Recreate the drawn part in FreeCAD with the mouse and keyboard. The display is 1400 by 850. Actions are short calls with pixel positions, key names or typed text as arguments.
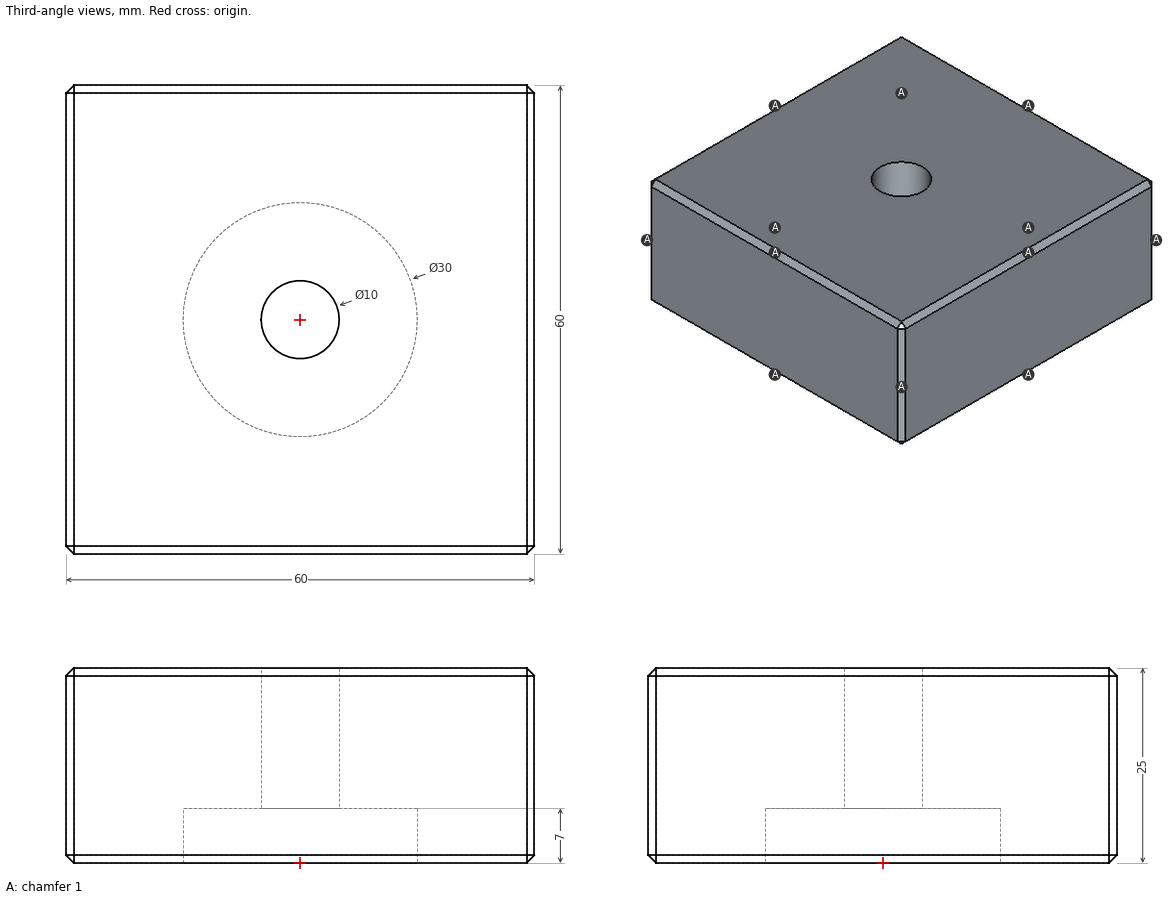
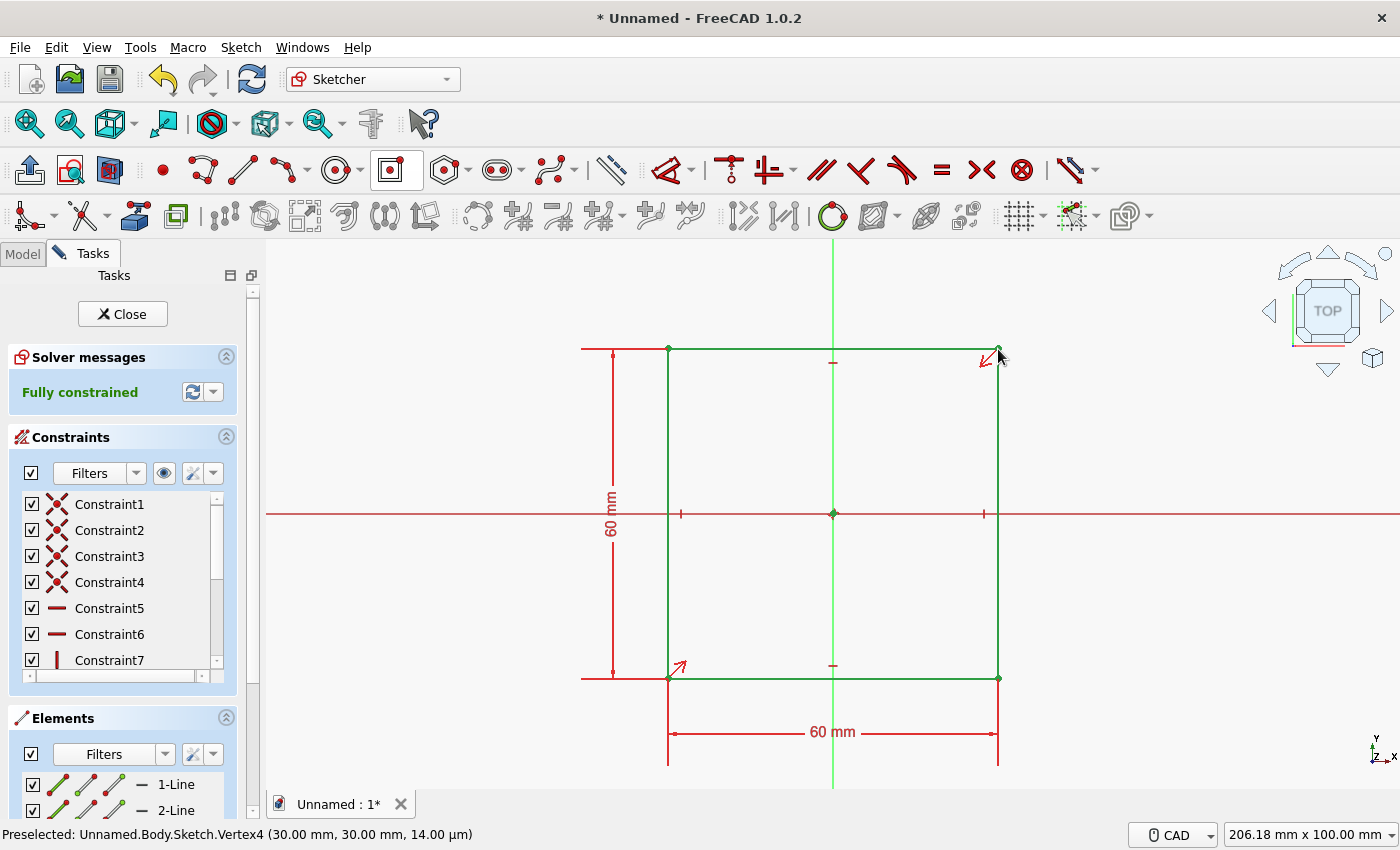
click(123, 314)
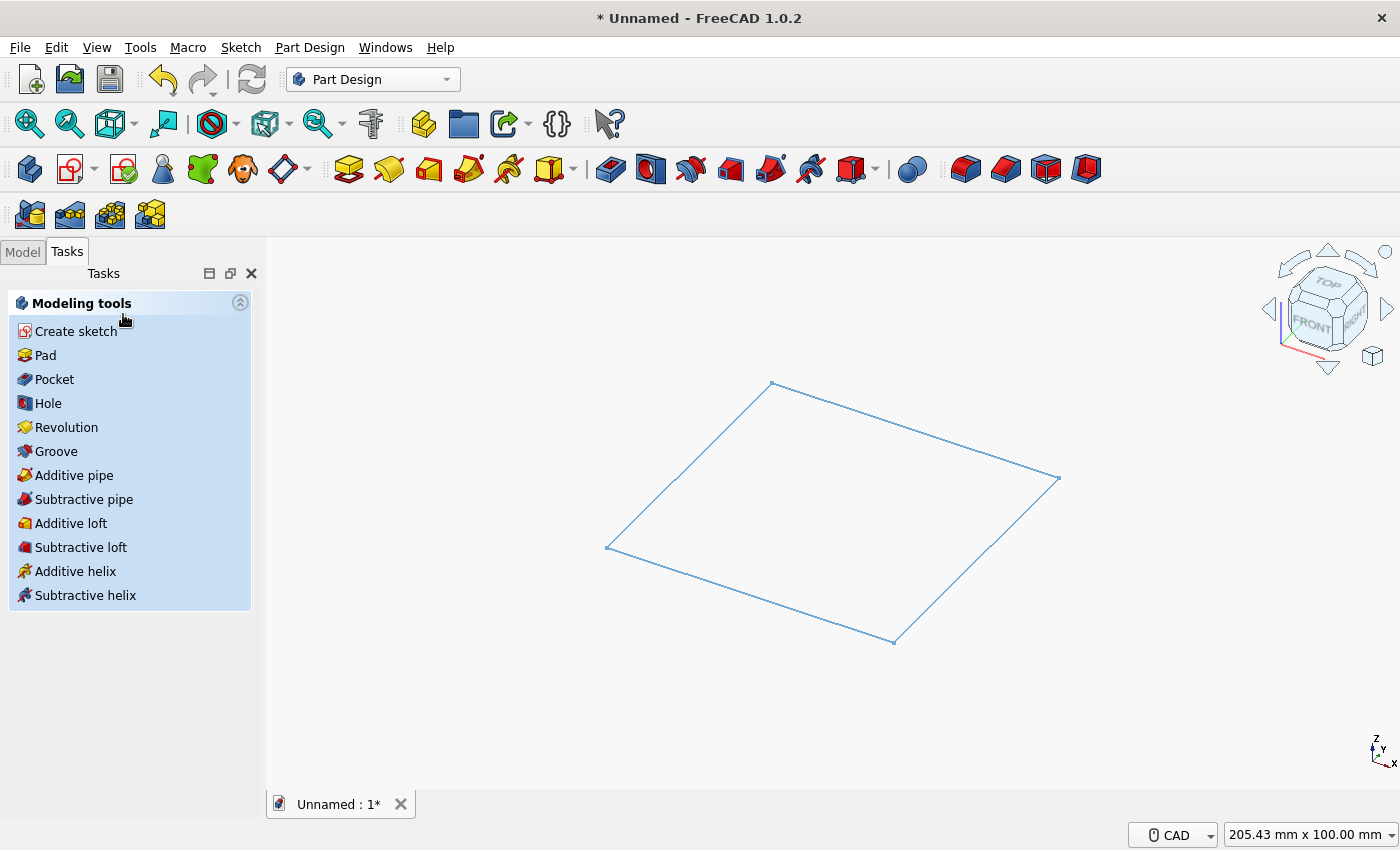
click(350, 170)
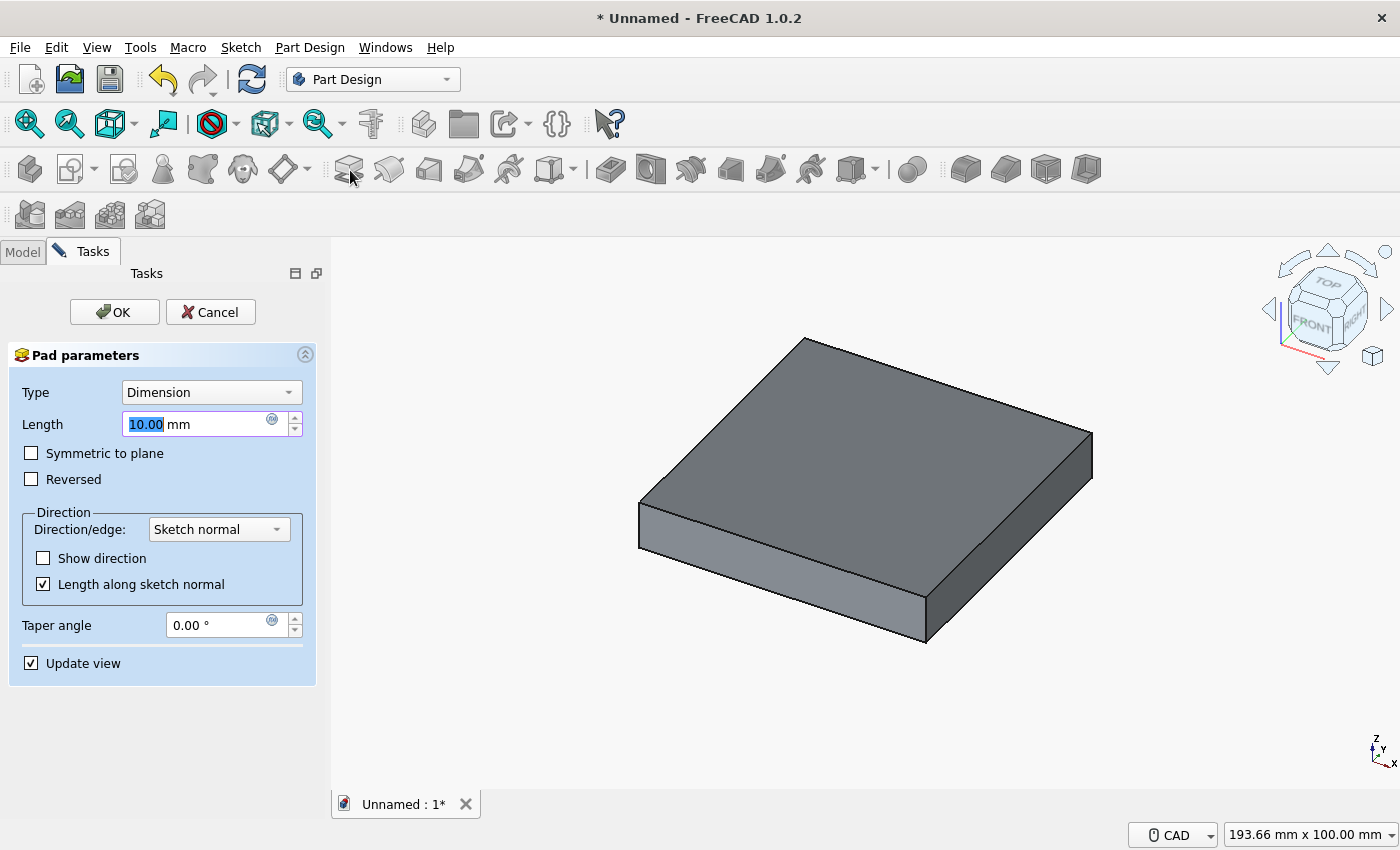
text(25)
key(Tab)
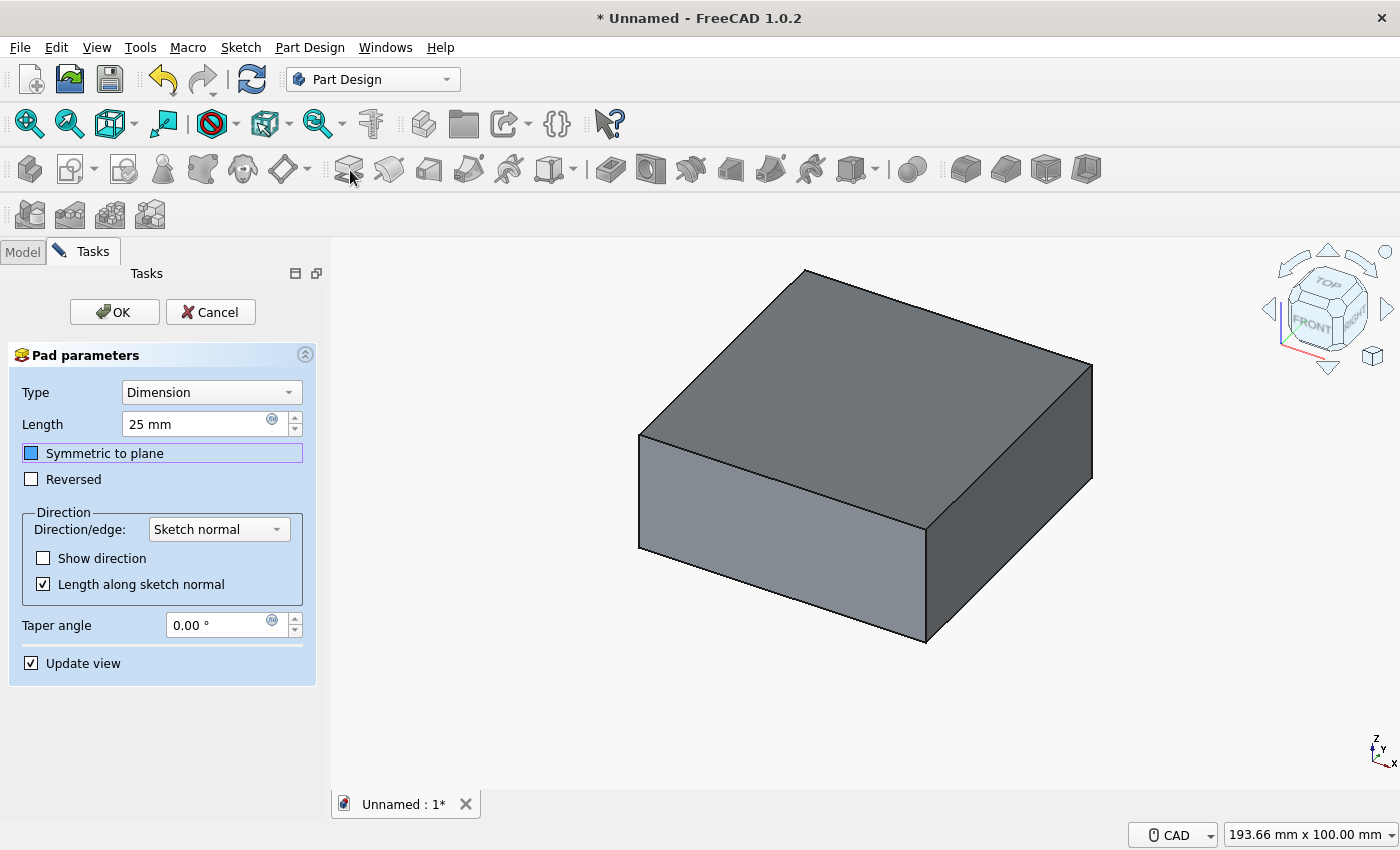
click(115, 312)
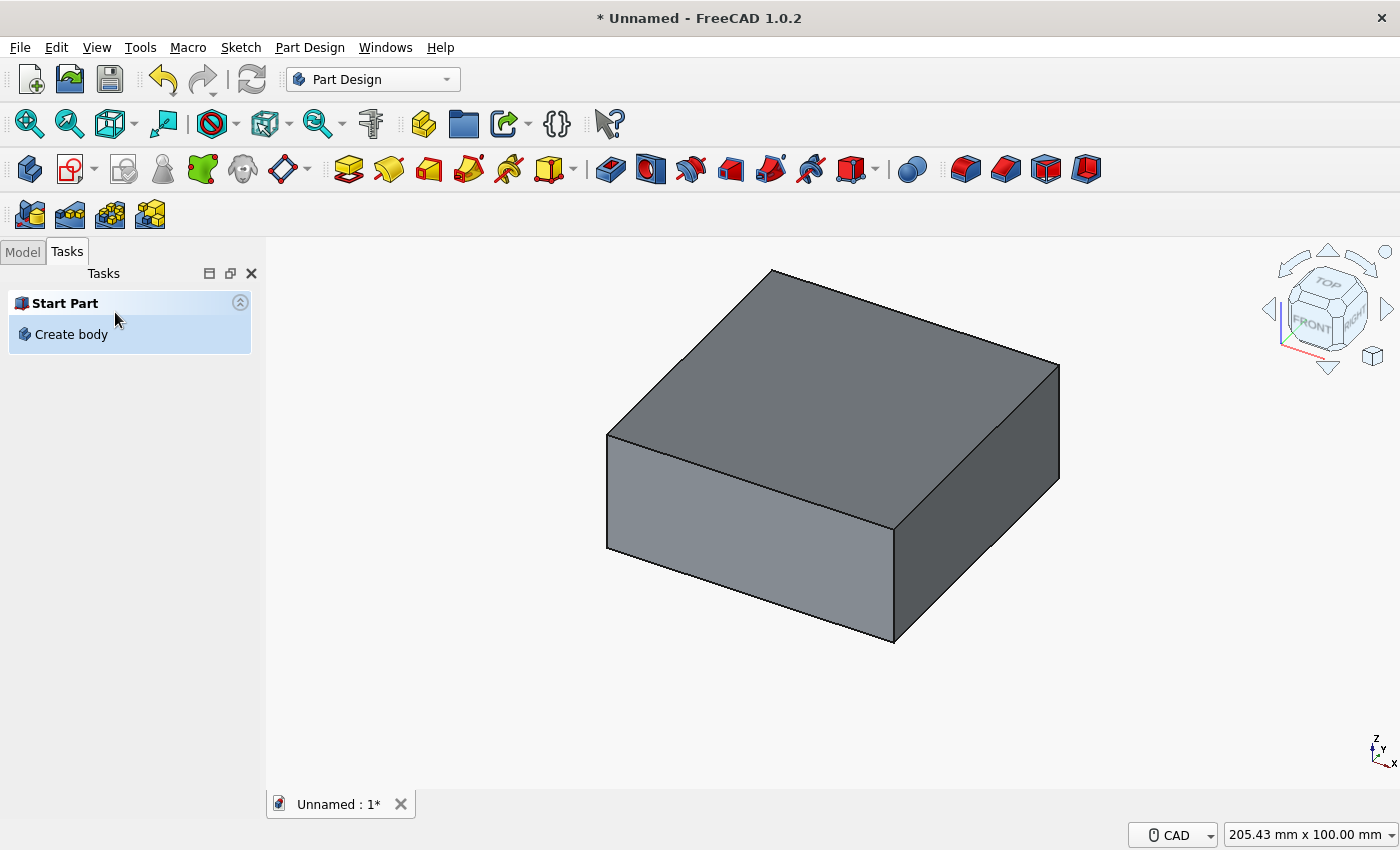
click(833, 399)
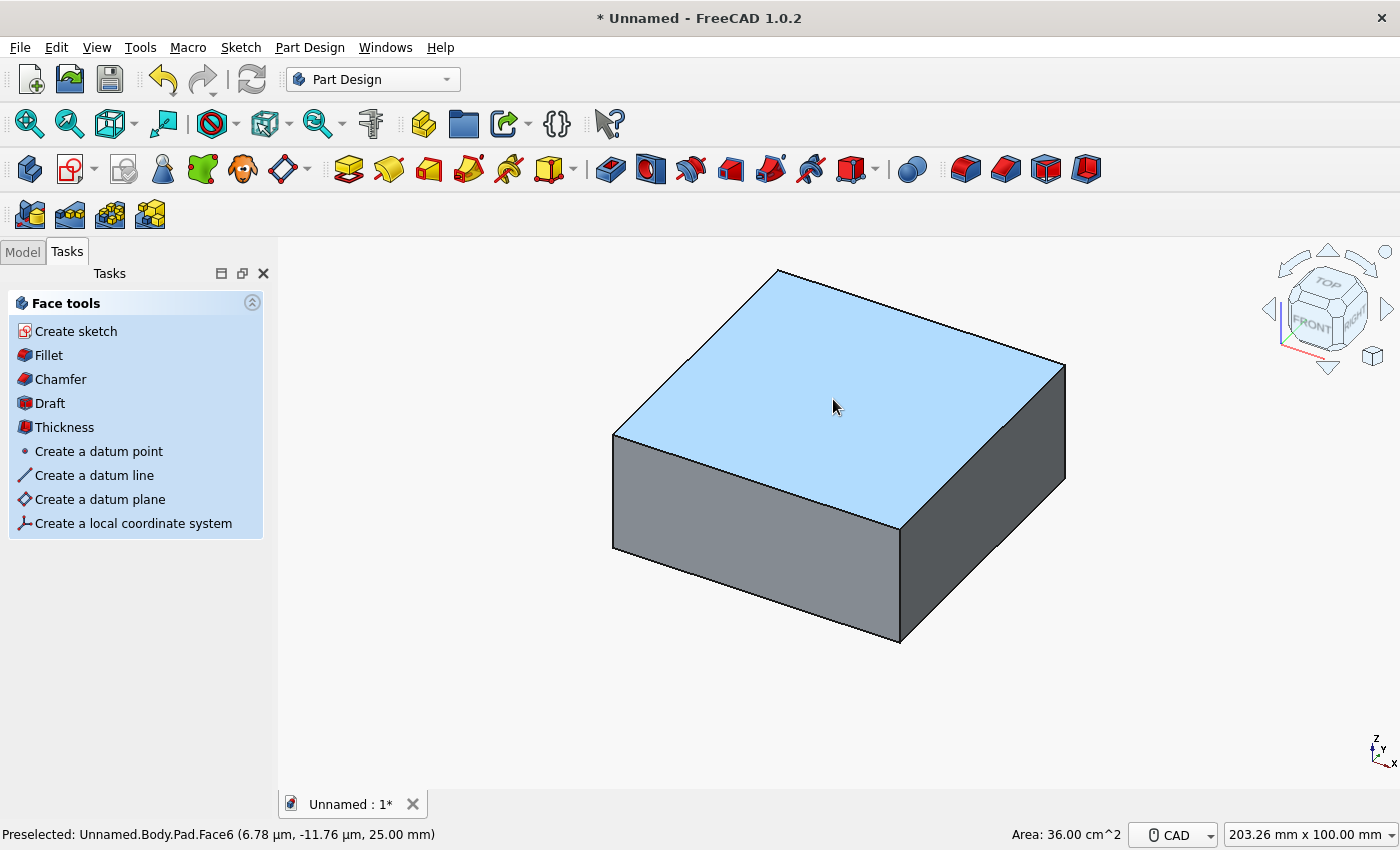
click(900, 585, ctrl)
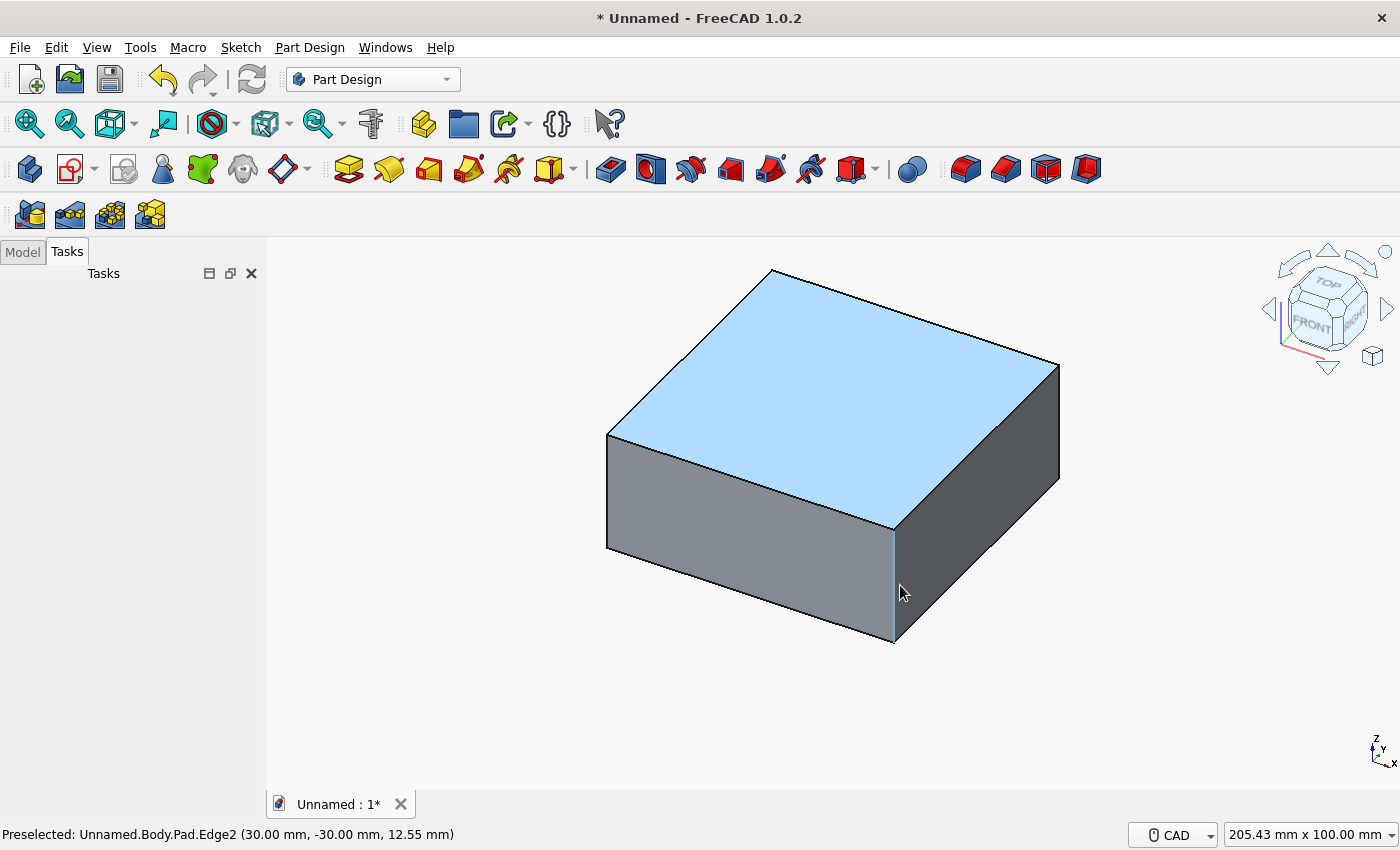
key(0)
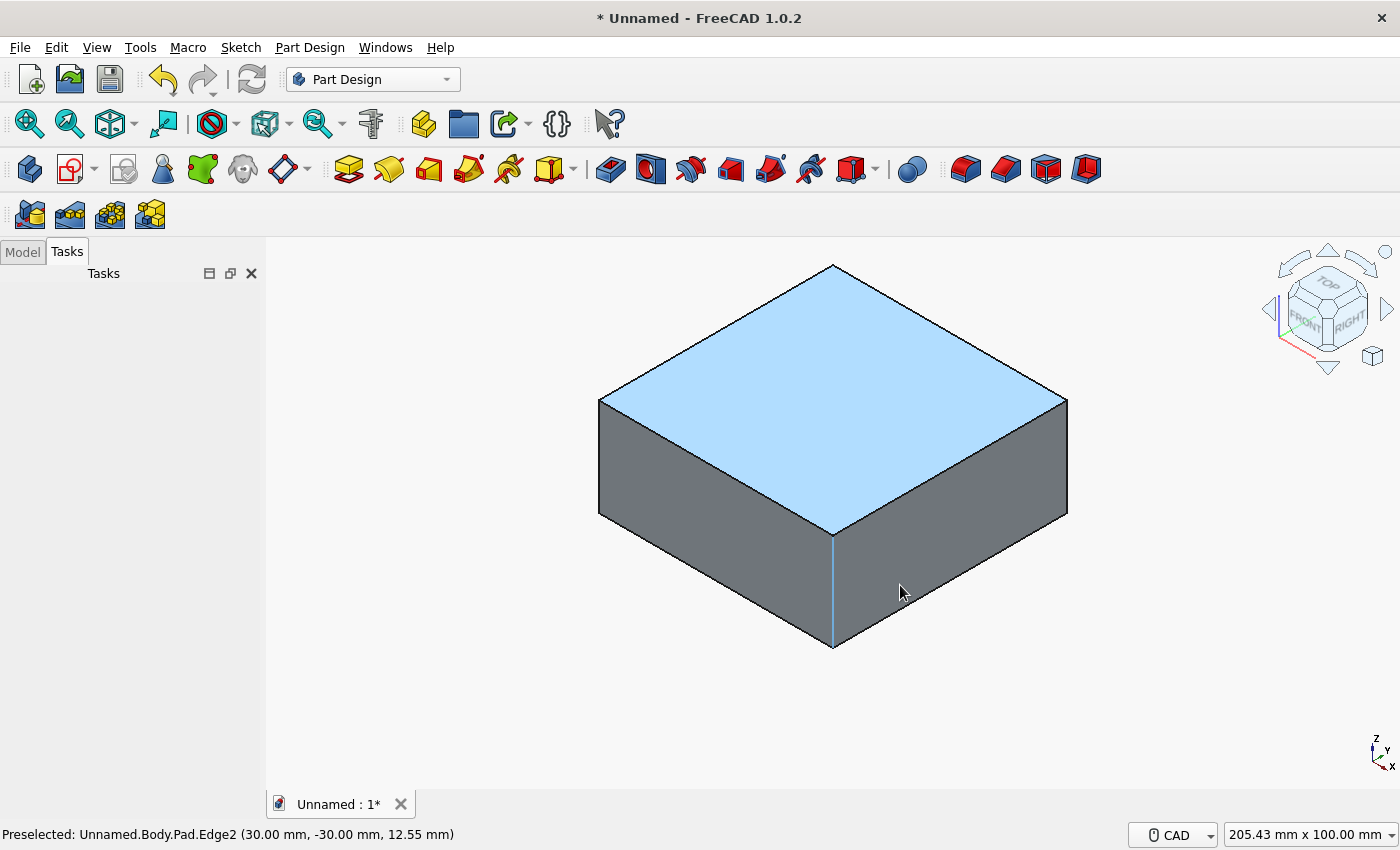
key(2)